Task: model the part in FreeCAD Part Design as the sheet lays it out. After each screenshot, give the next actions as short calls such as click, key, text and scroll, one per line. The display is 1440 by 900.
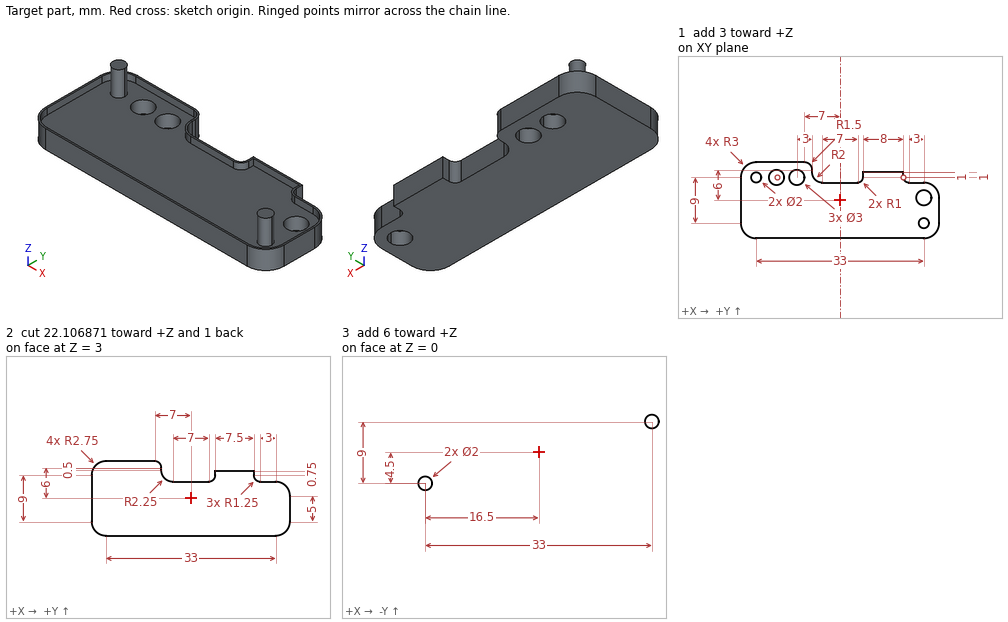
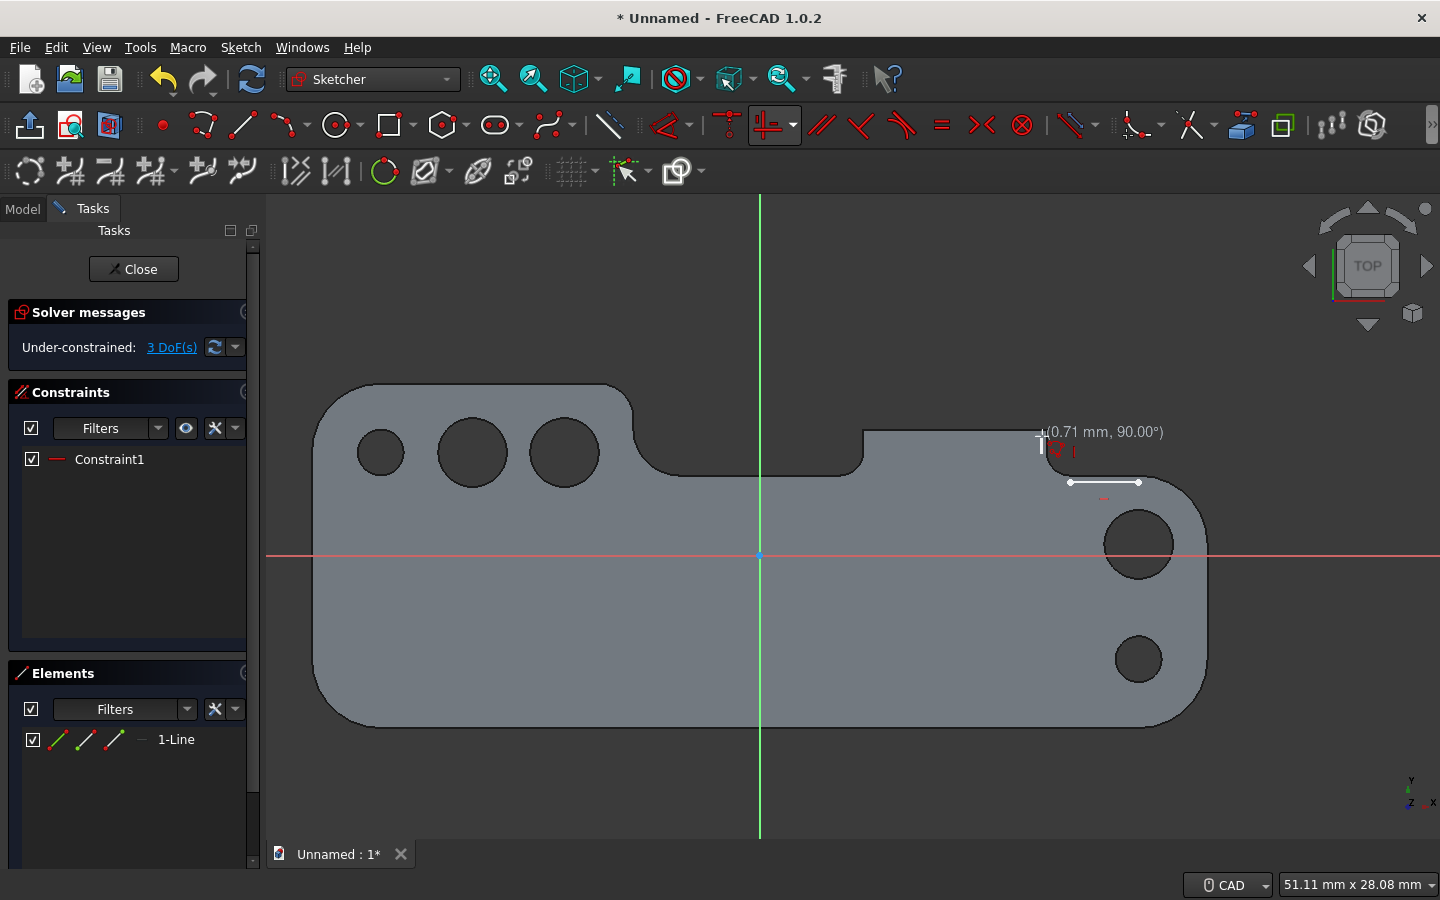
click(1042, 435)
click(869, 435)
click(869, 453)
right_click(869, 453)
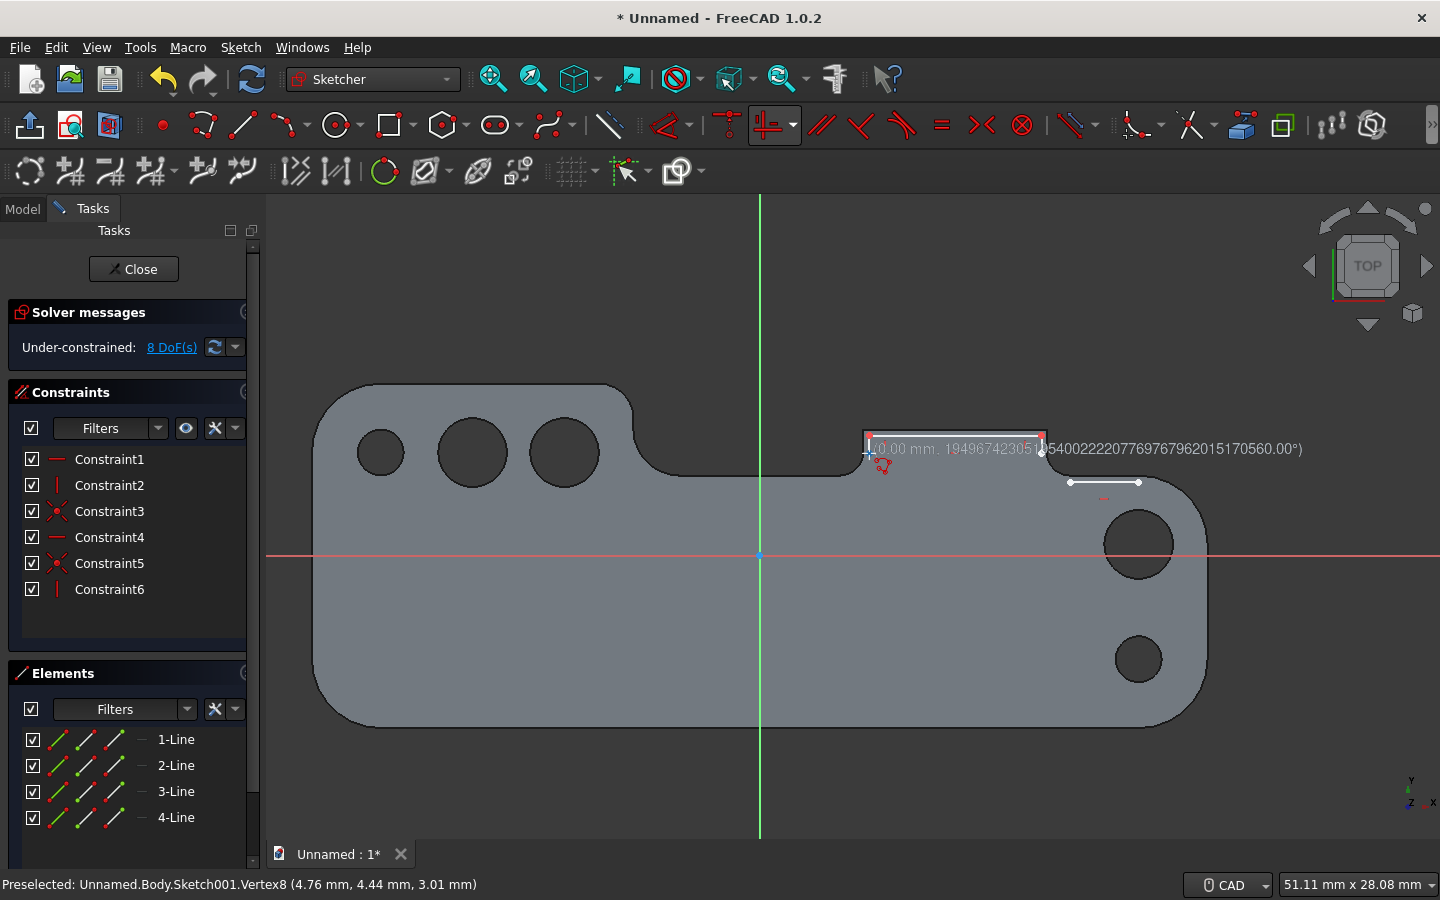
click(244, 126)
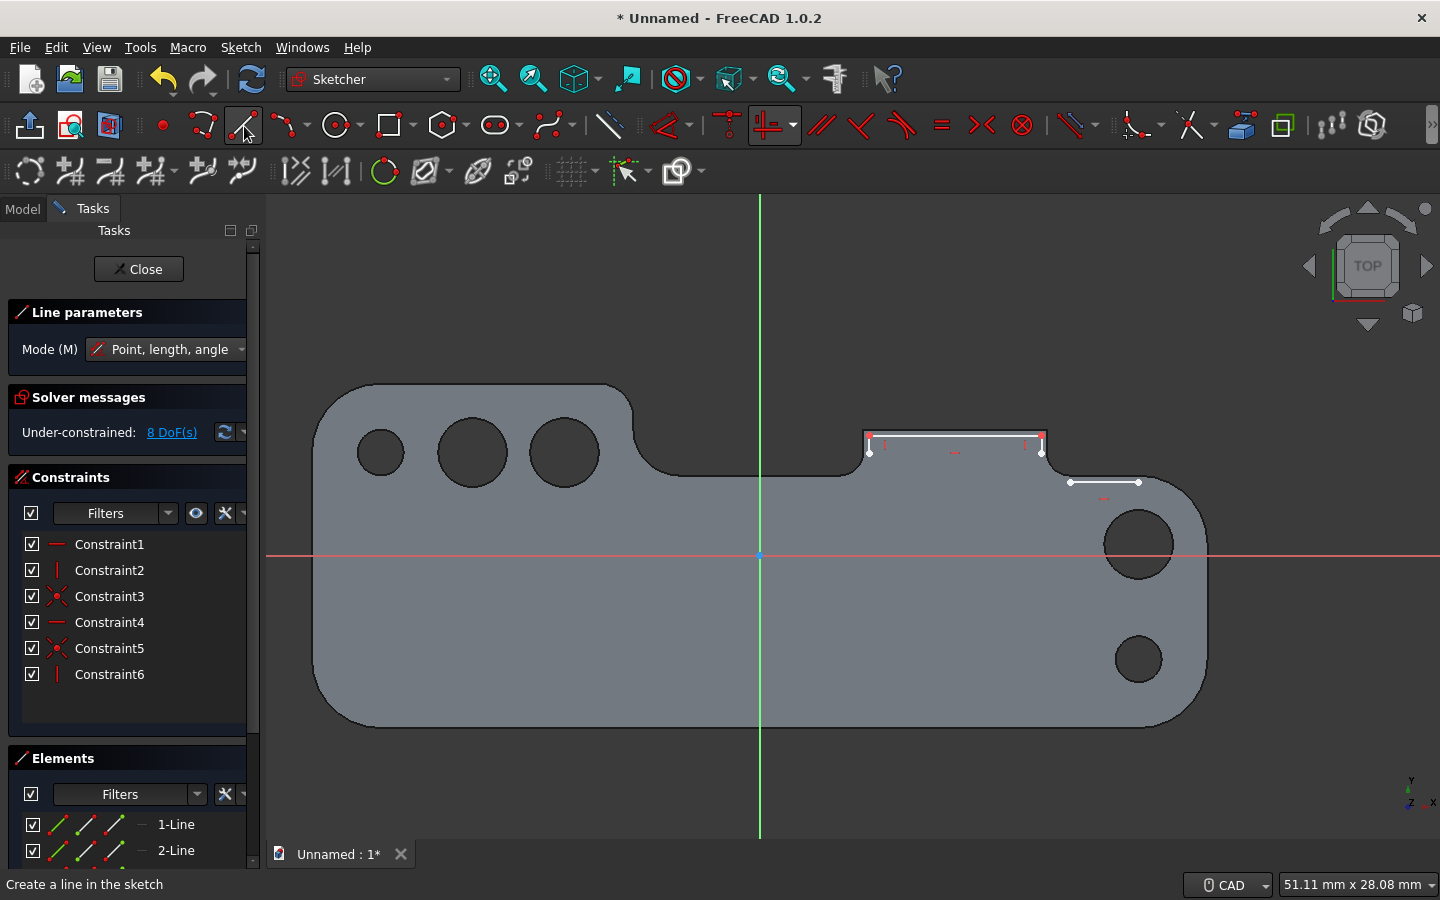
click(840, 481)
click(679, 481)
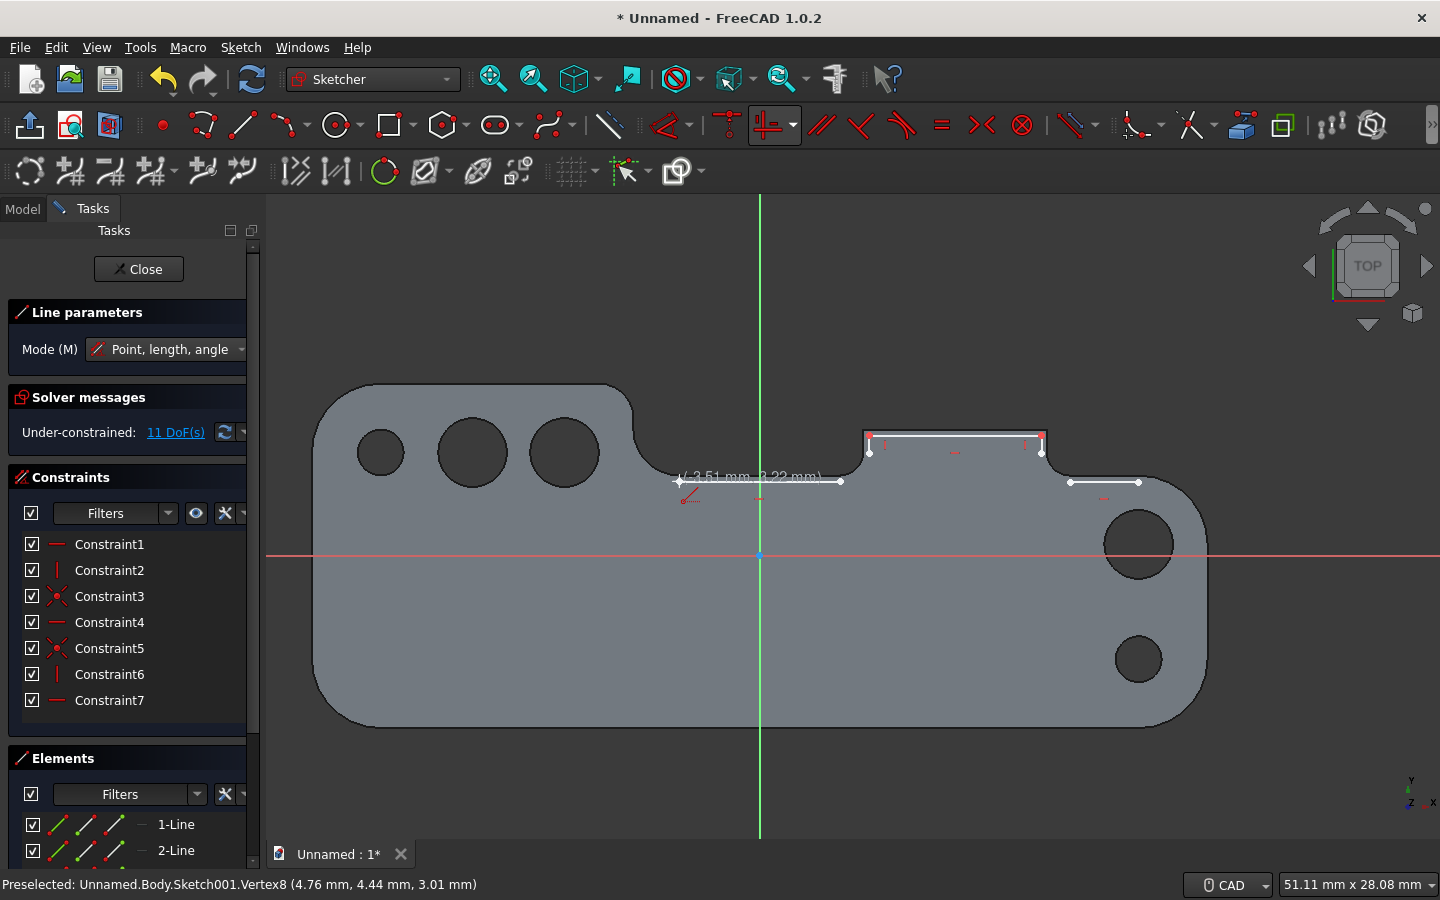
click(628, 430)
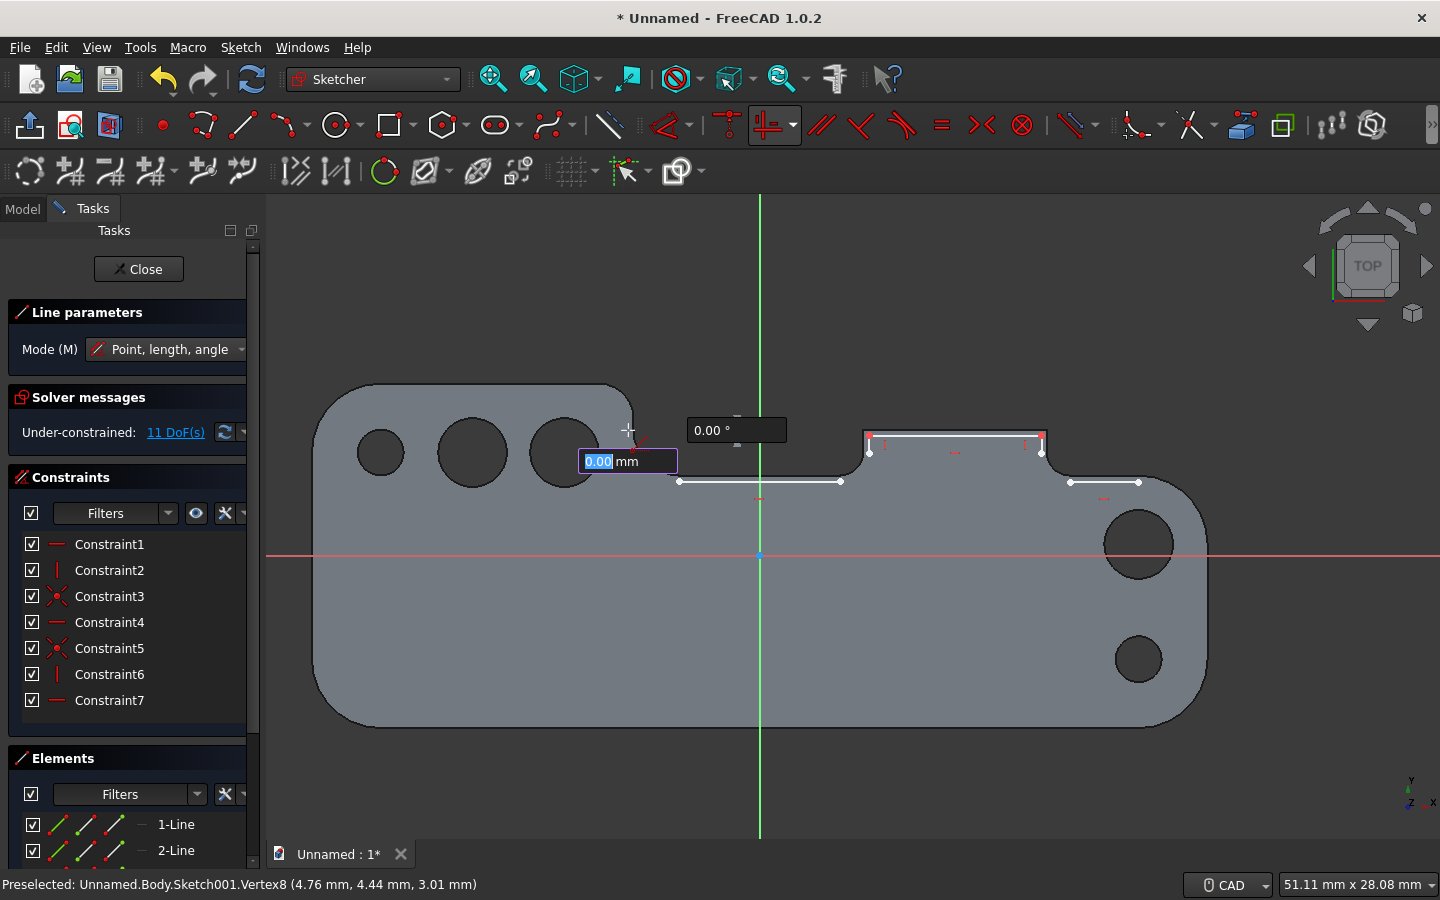
scroll(628, 418, up, 2)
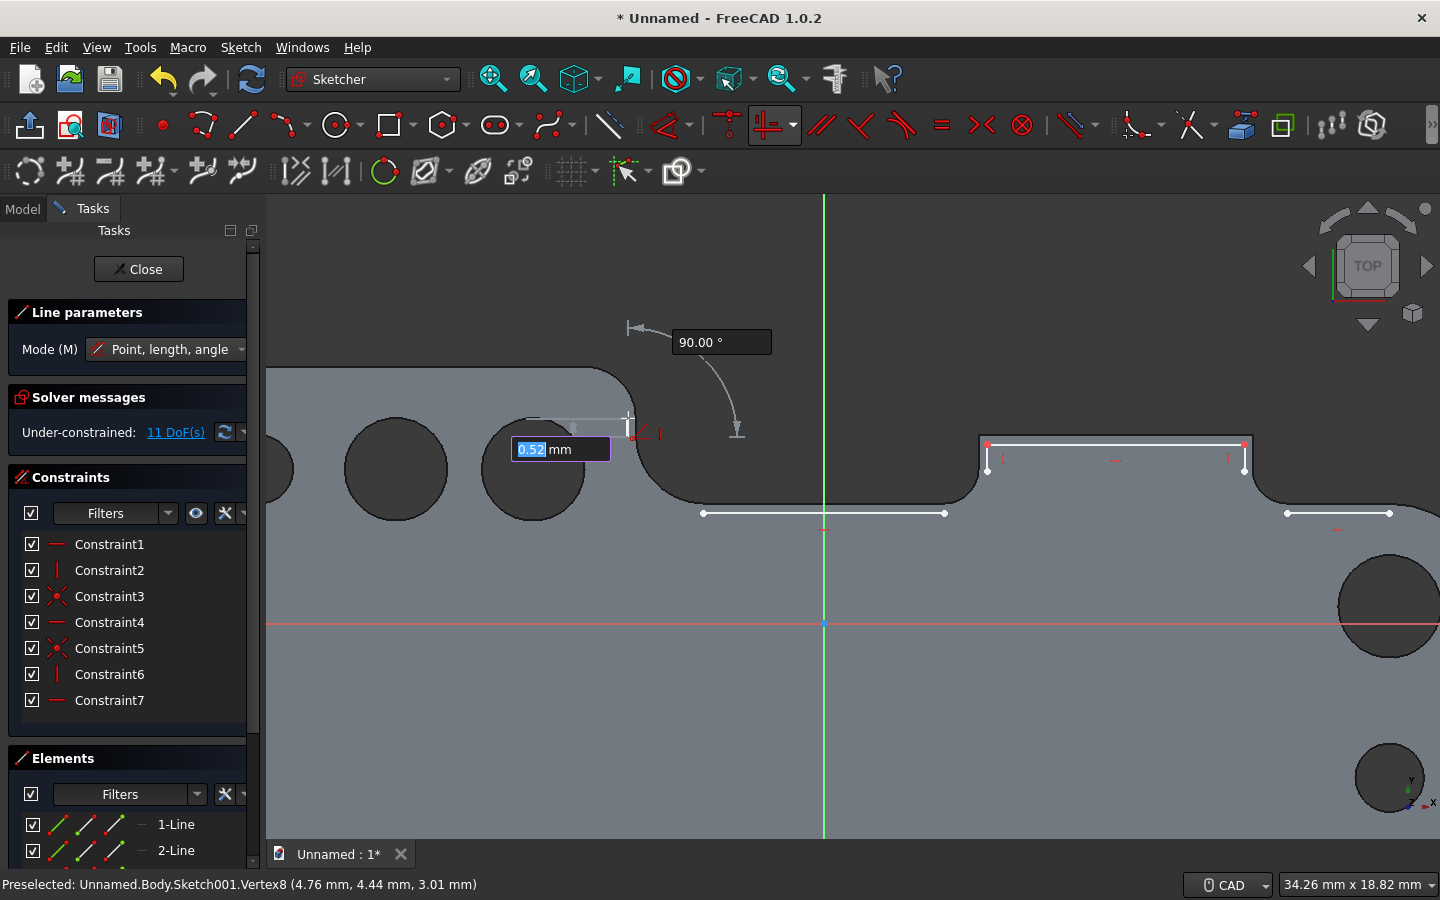
click(628, 418)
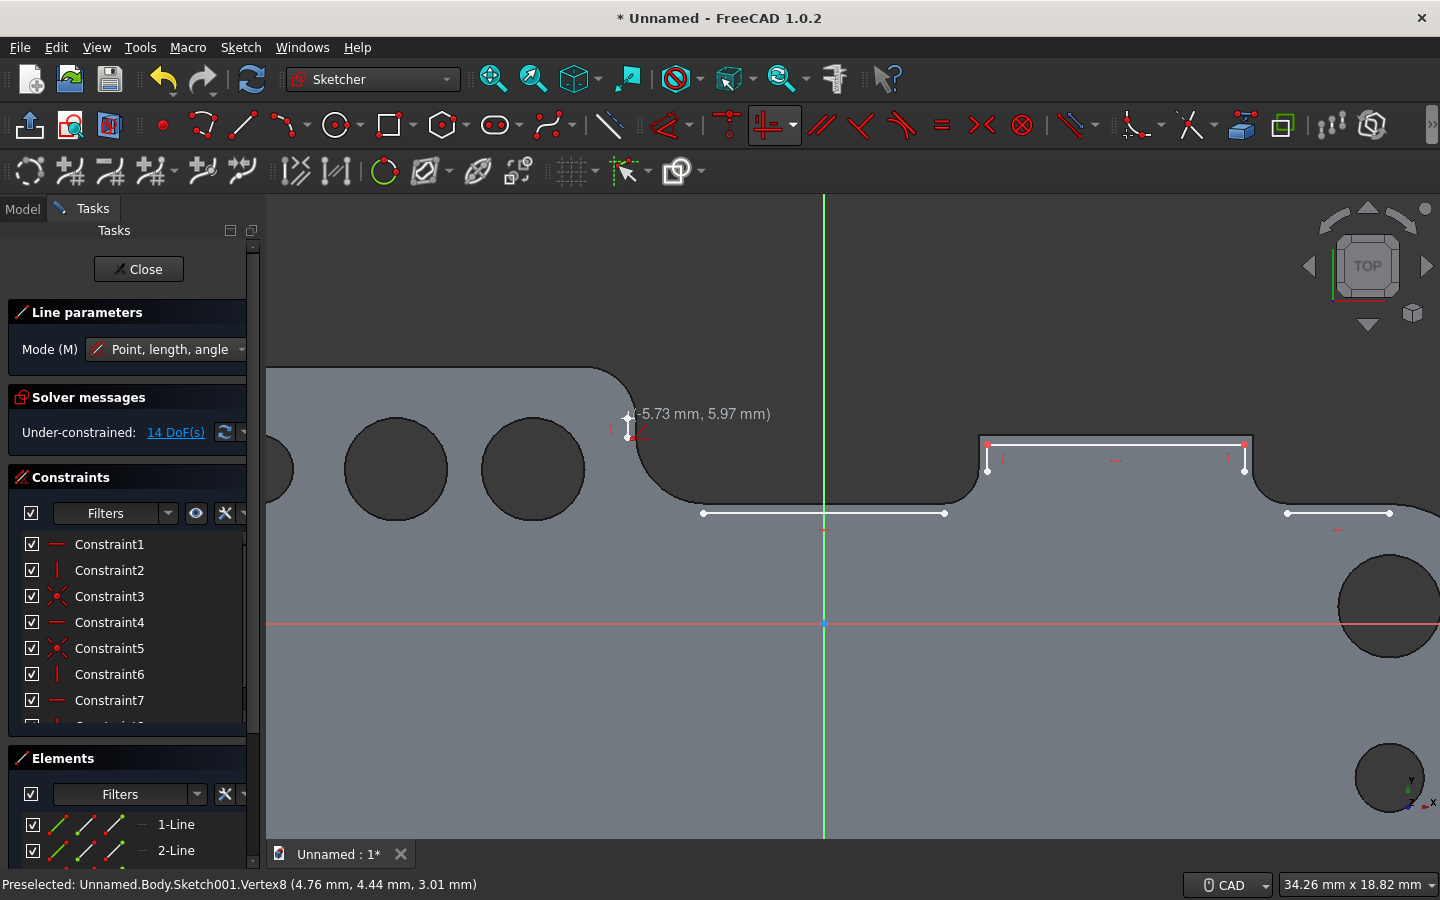
click(584, 375)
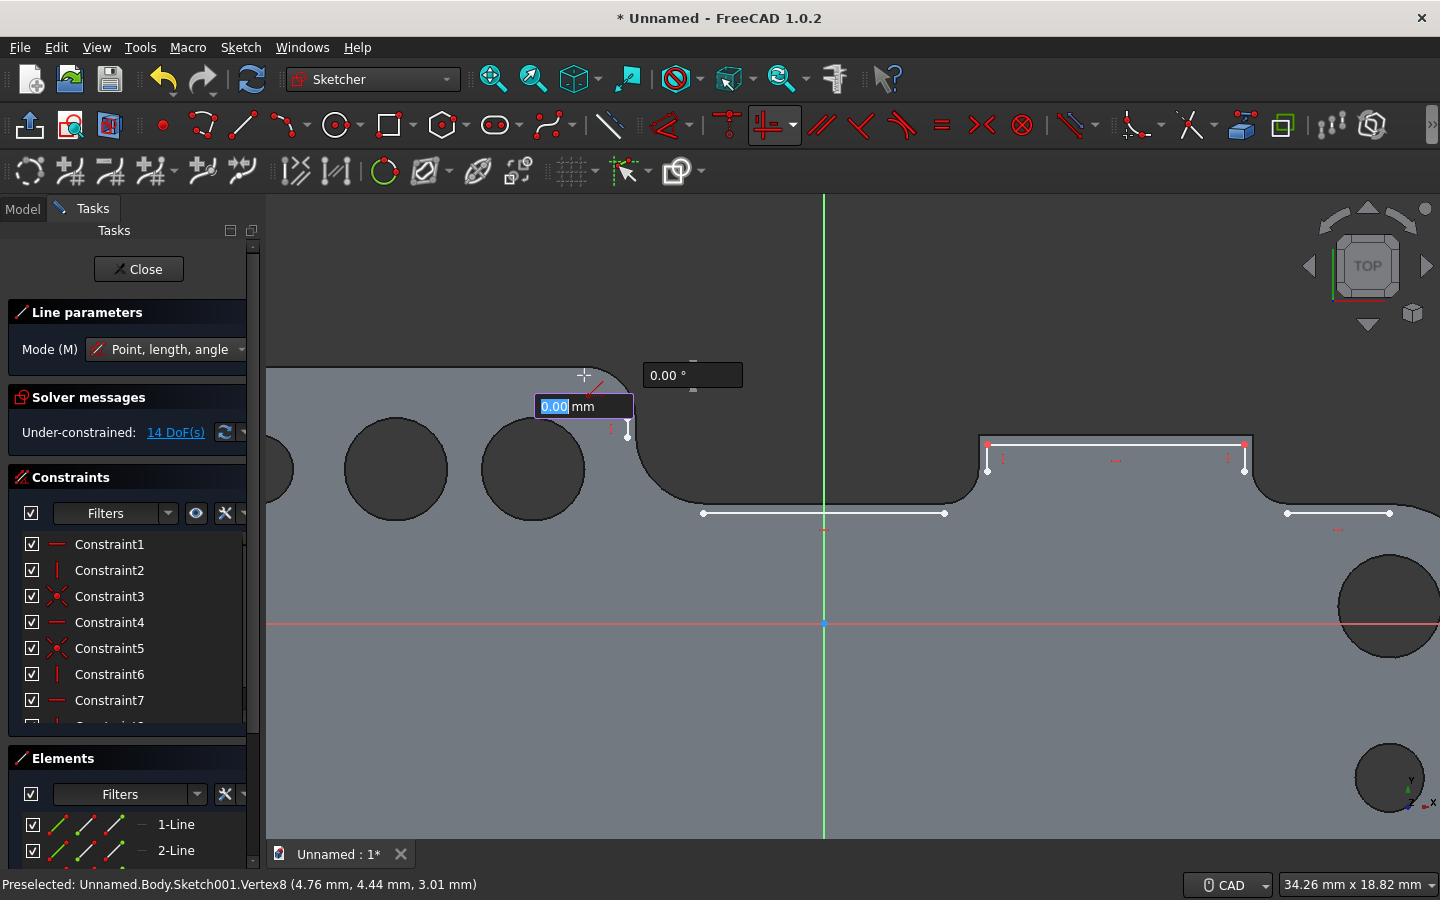
scroll(736, 386, down, 3)